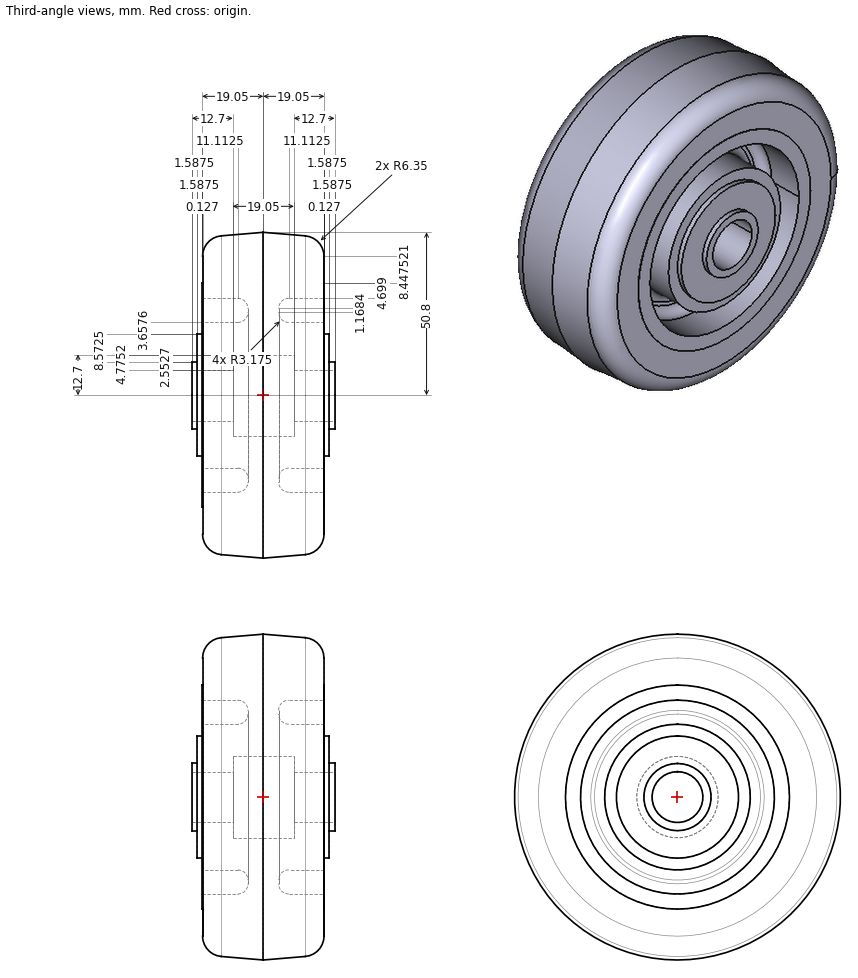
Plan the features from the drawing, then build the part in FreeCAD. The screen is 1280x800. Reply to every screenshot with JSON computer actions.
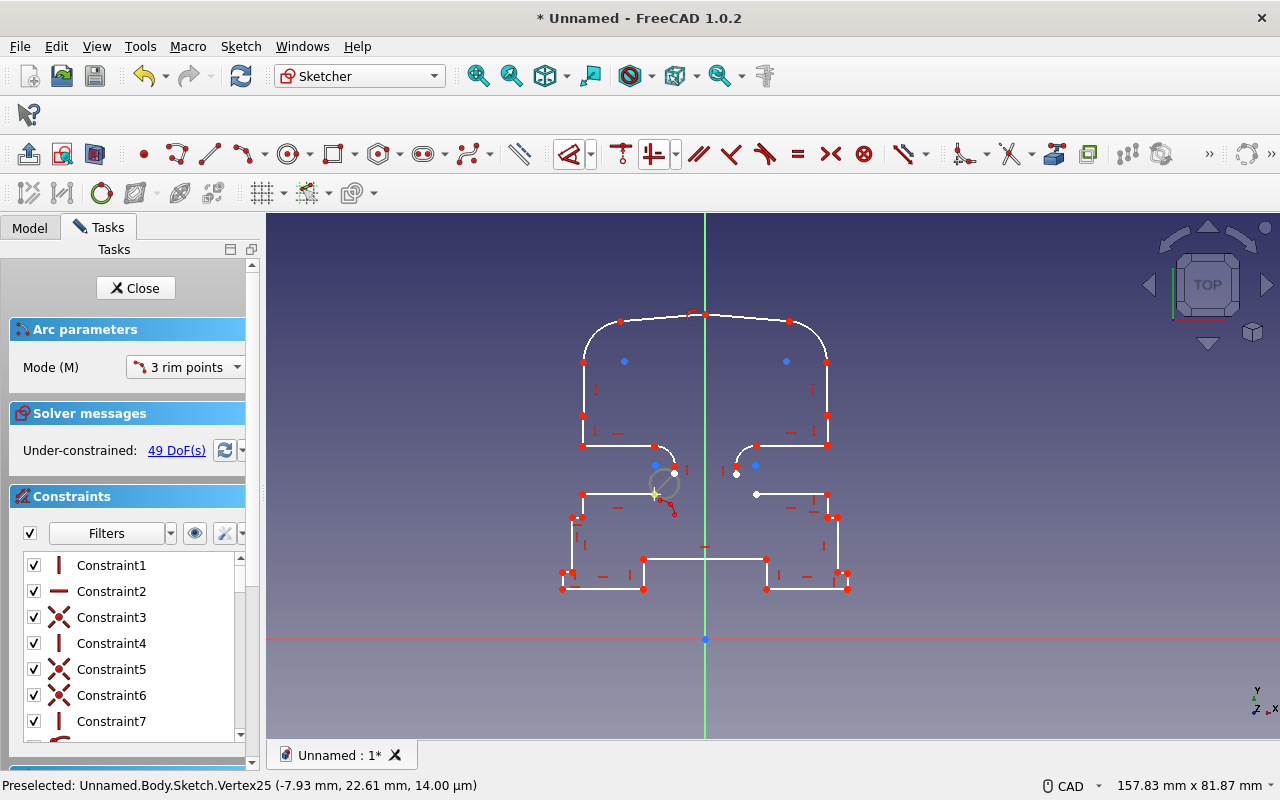
{"action": "scroll", "coordinate": [669, 488], "scroll_direction": "up", "scroll_amount": 5}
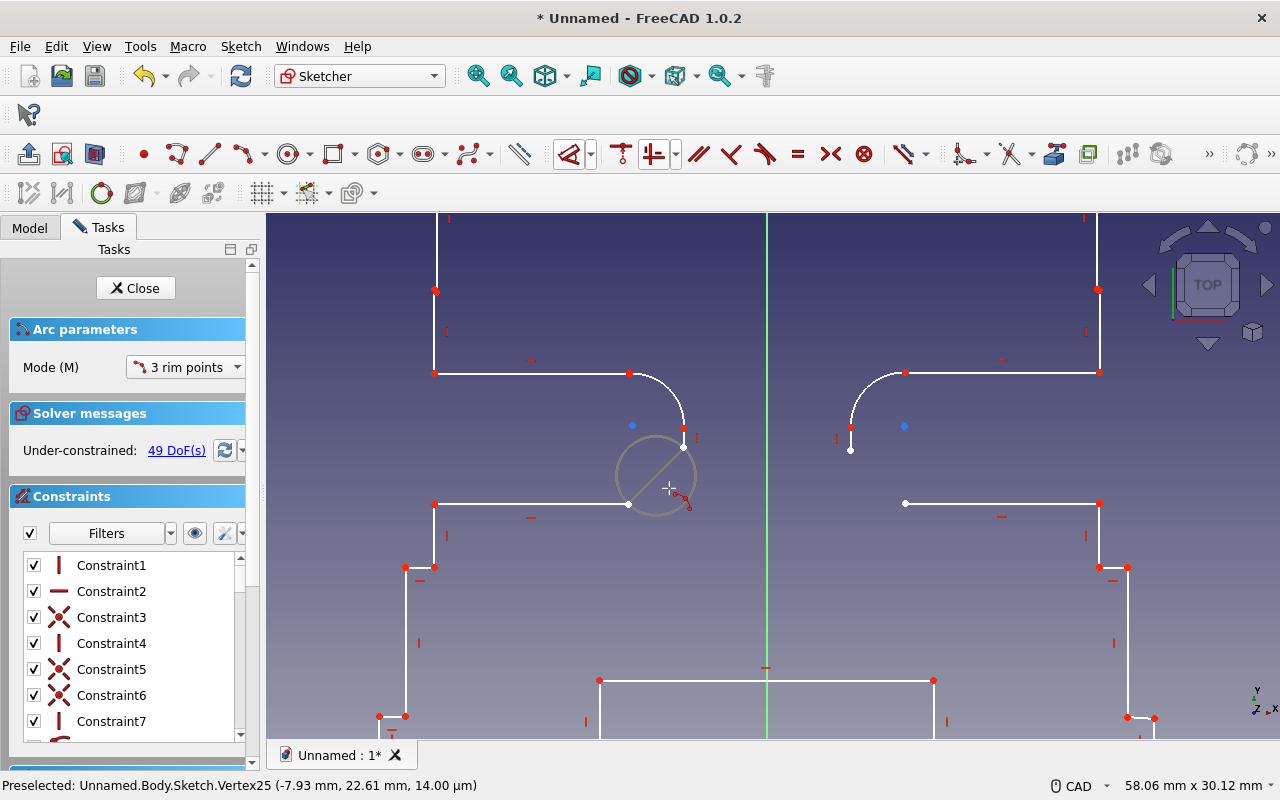
{"action": "left_click", "coordinate": [667, 486]}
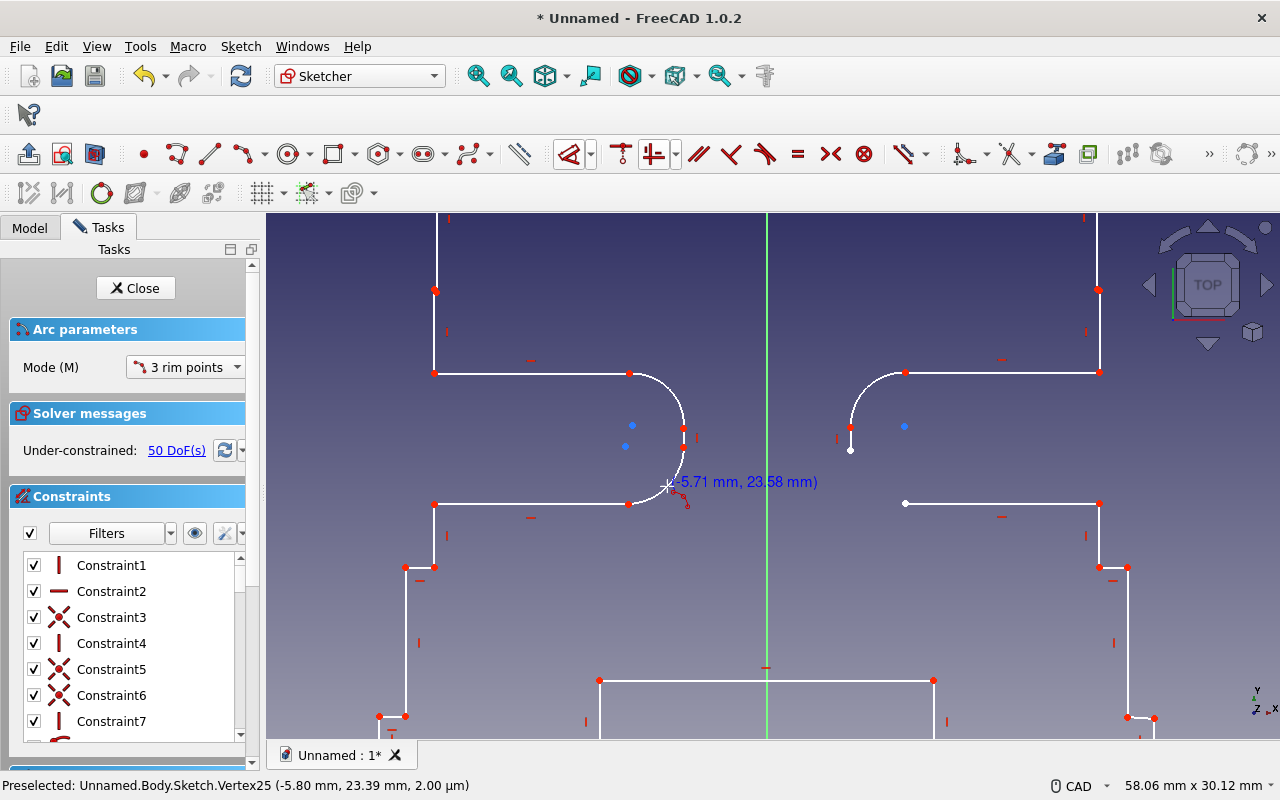
{"action": "left_click", "coordinate": [905, 504]}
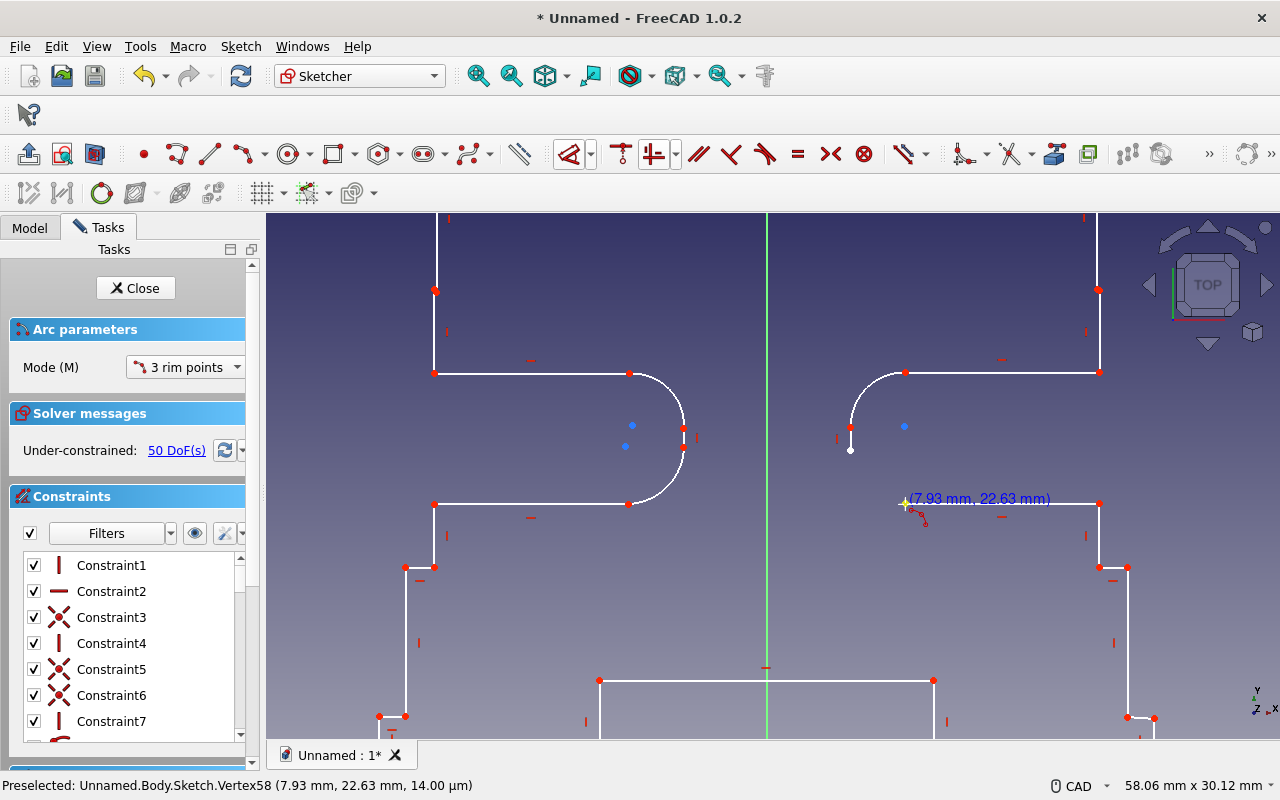
{"action": "scroll", "coordinate": [850, 447], "scroll_direction": "up", "scroll_amount": 3}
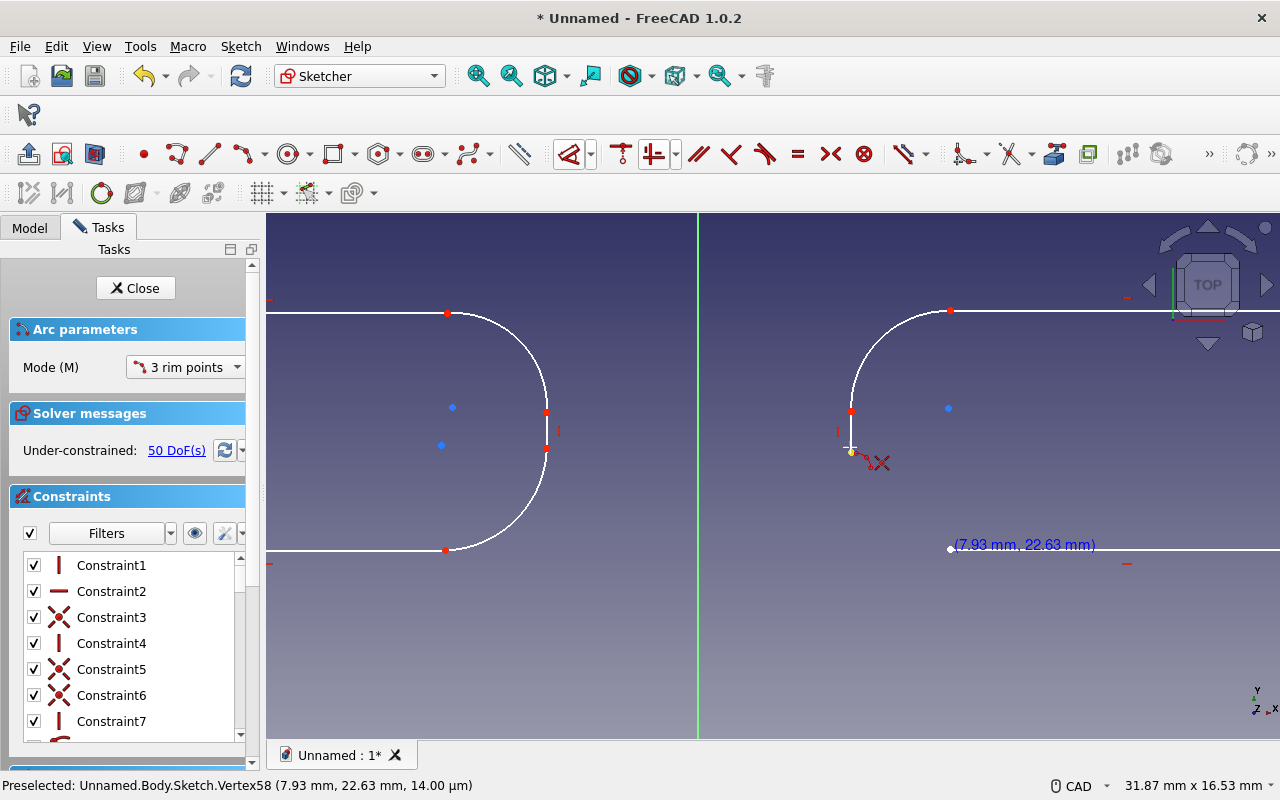
{"action": "left_click", "coordinate": [851, 452]}
{"action": "left_click", "coordinate": [879, 518]}
{"action": "key", "text": "Escape"}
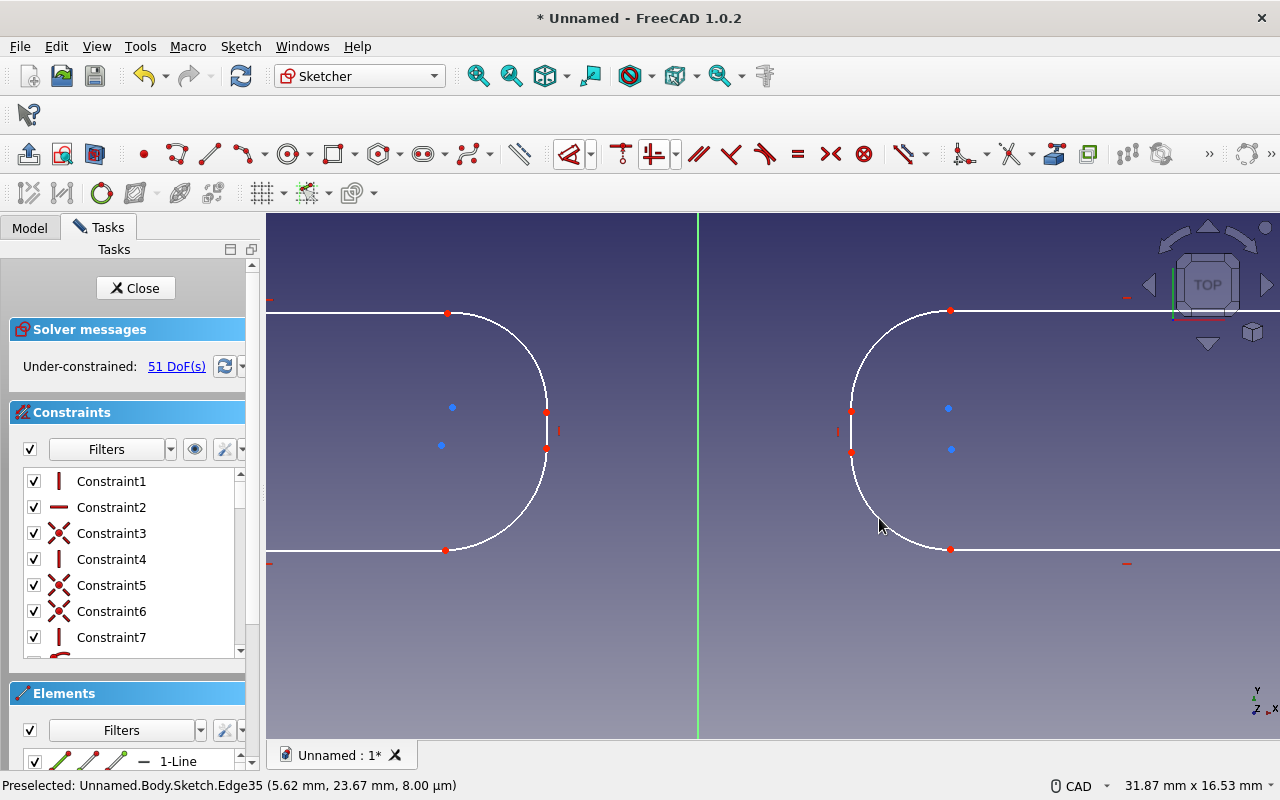
{"action": "left_click", "coordinate": [851, 440]}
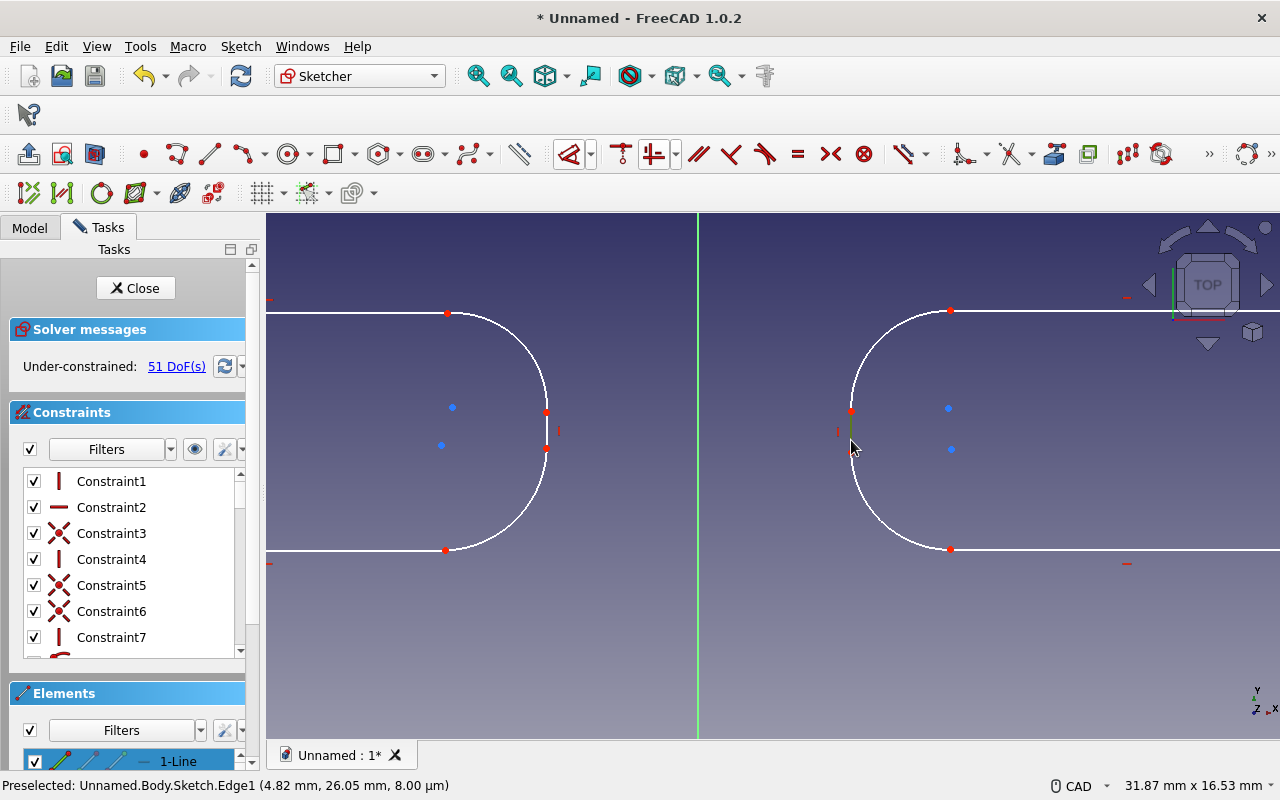
{"action": "scroll", "coordinate": [706, 480], "scroll_direction": "down", "scroll_amount": 8}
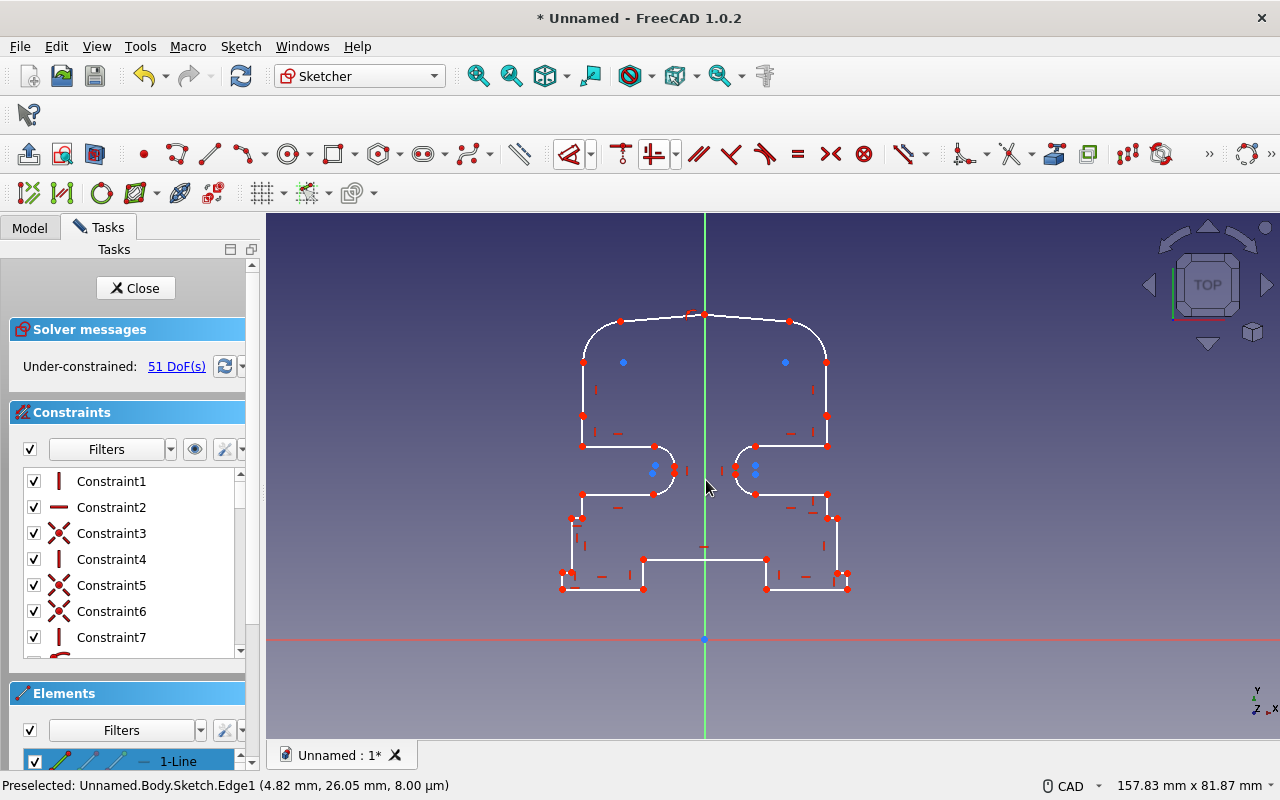
{"action": "scroll", "coordinate": [746, 448], "scroll_direction": "up", "scroll_amount": 2}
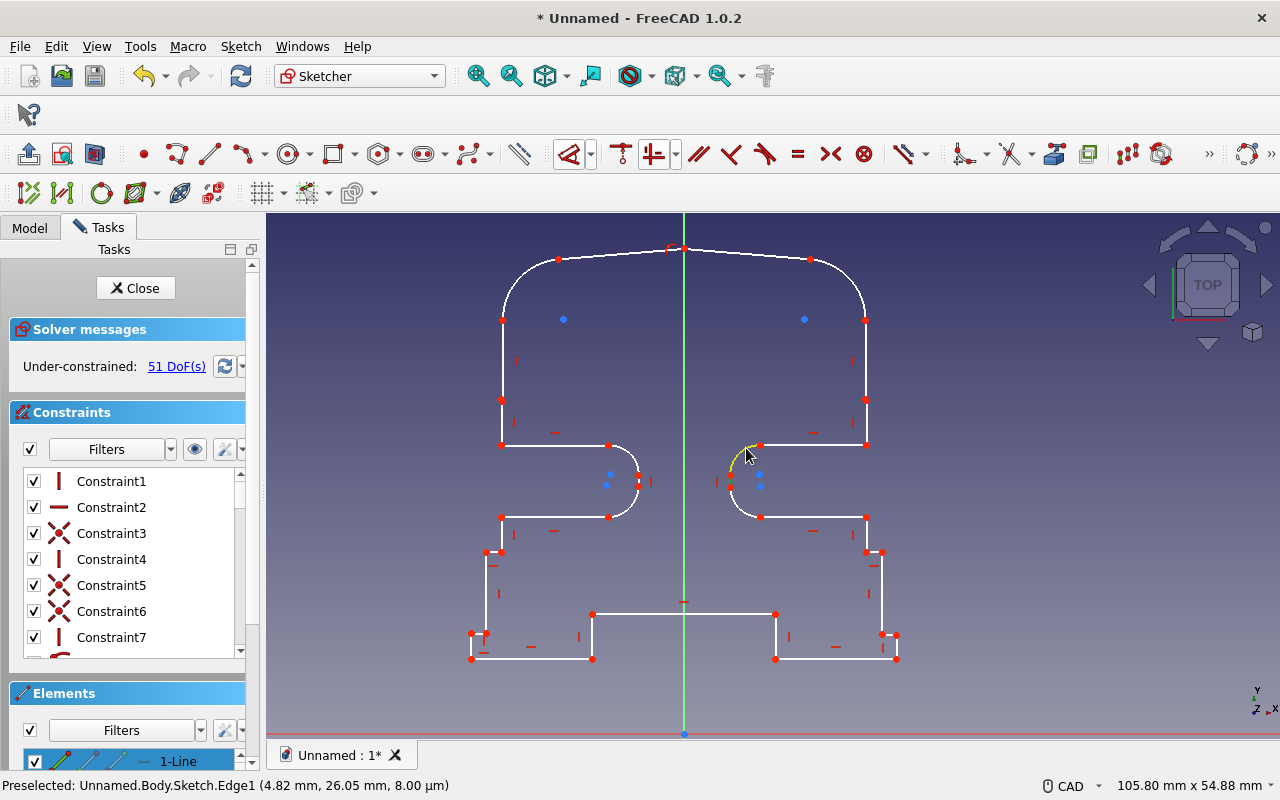
{"action": "left_click", "coordinate": [746, 448]}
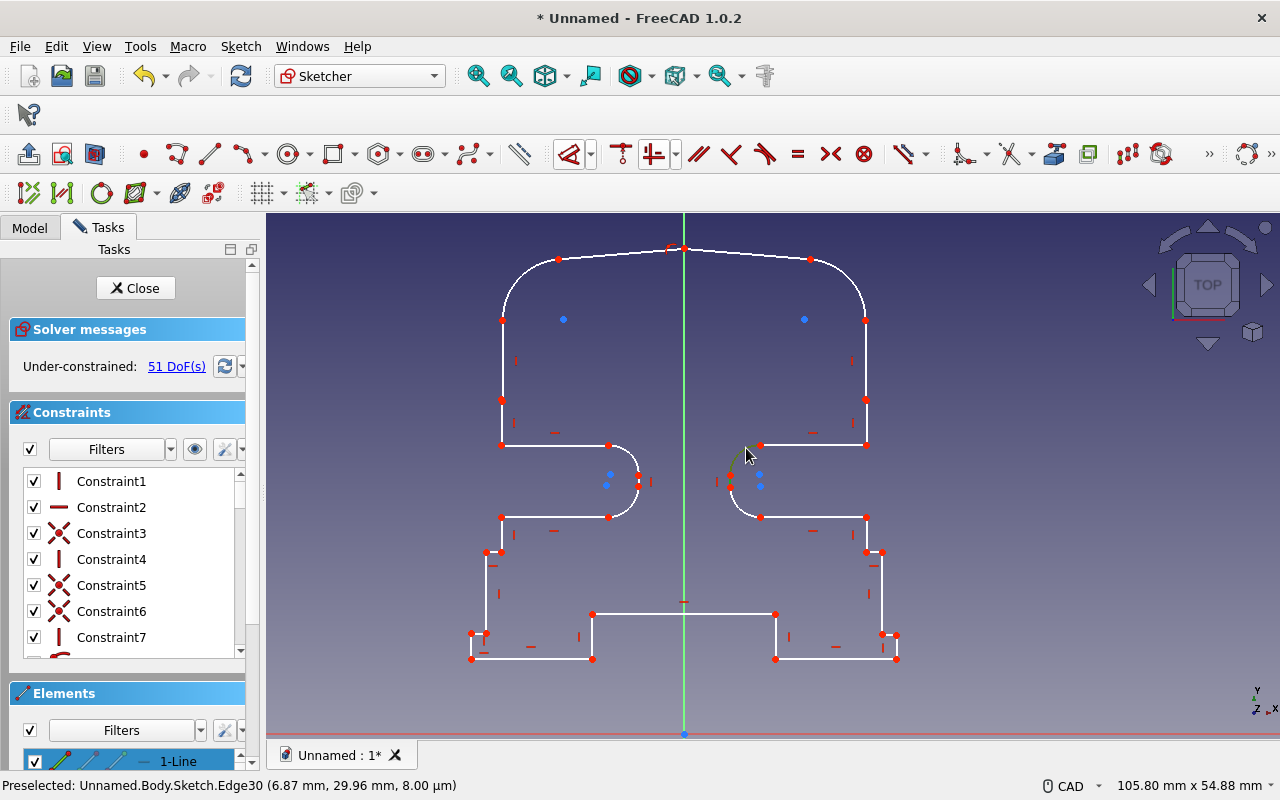
{"action": "left_click", "coordinate": [765, 154]}